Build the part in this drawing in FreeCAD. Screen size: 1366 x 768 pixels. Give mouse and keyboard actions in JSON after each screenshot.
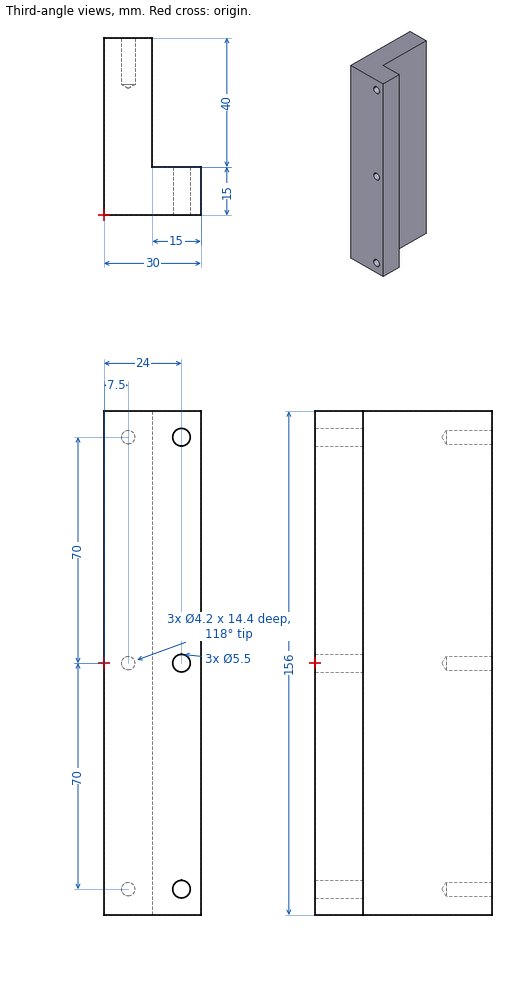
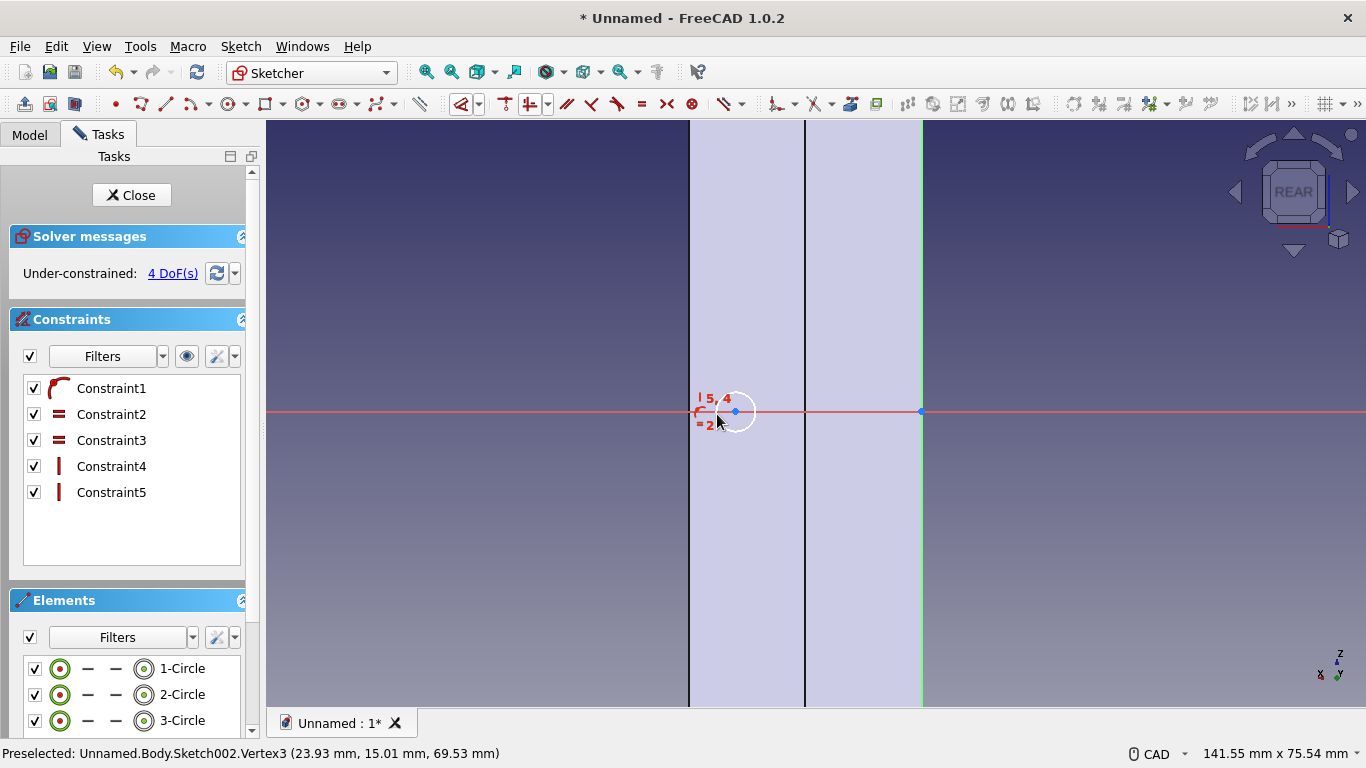
{"action": "left_click", "coordinate": [756, 413]}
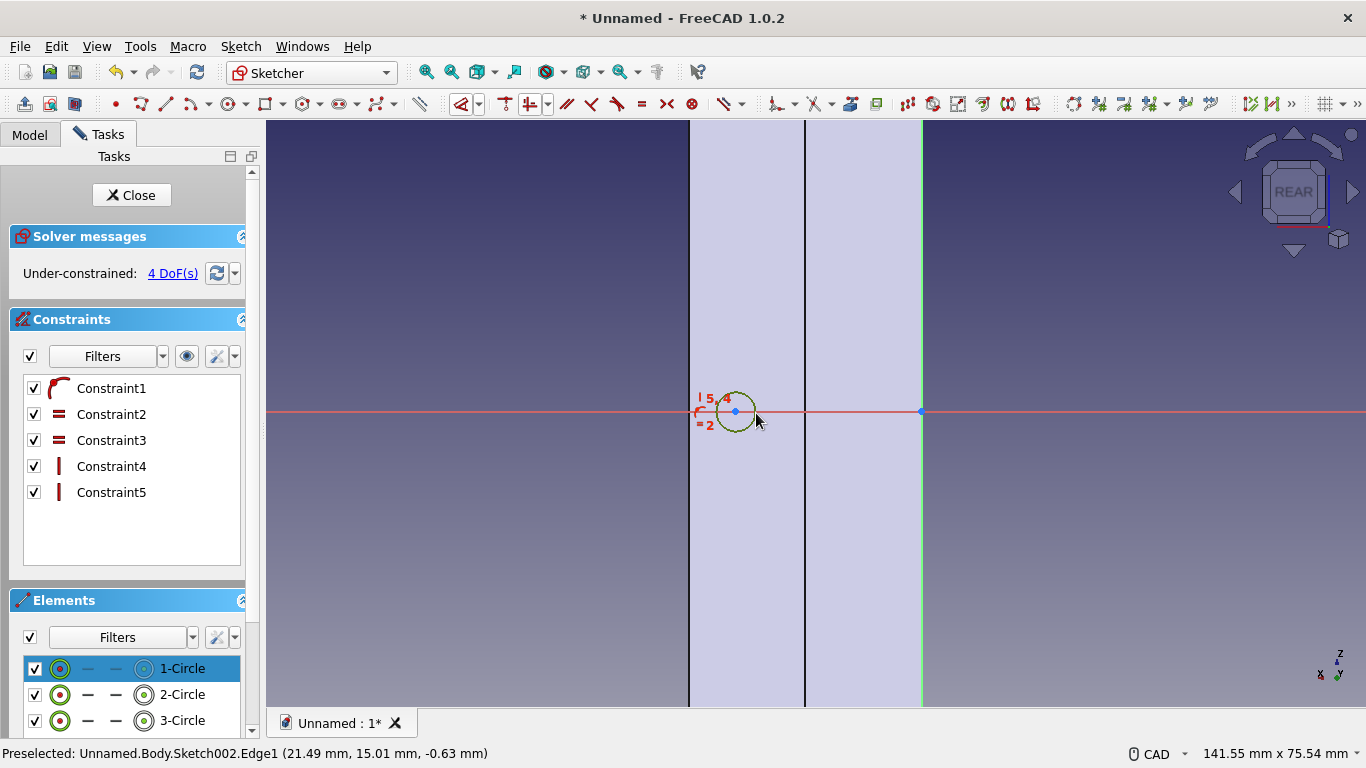
{"action": "key", "text": "k o"}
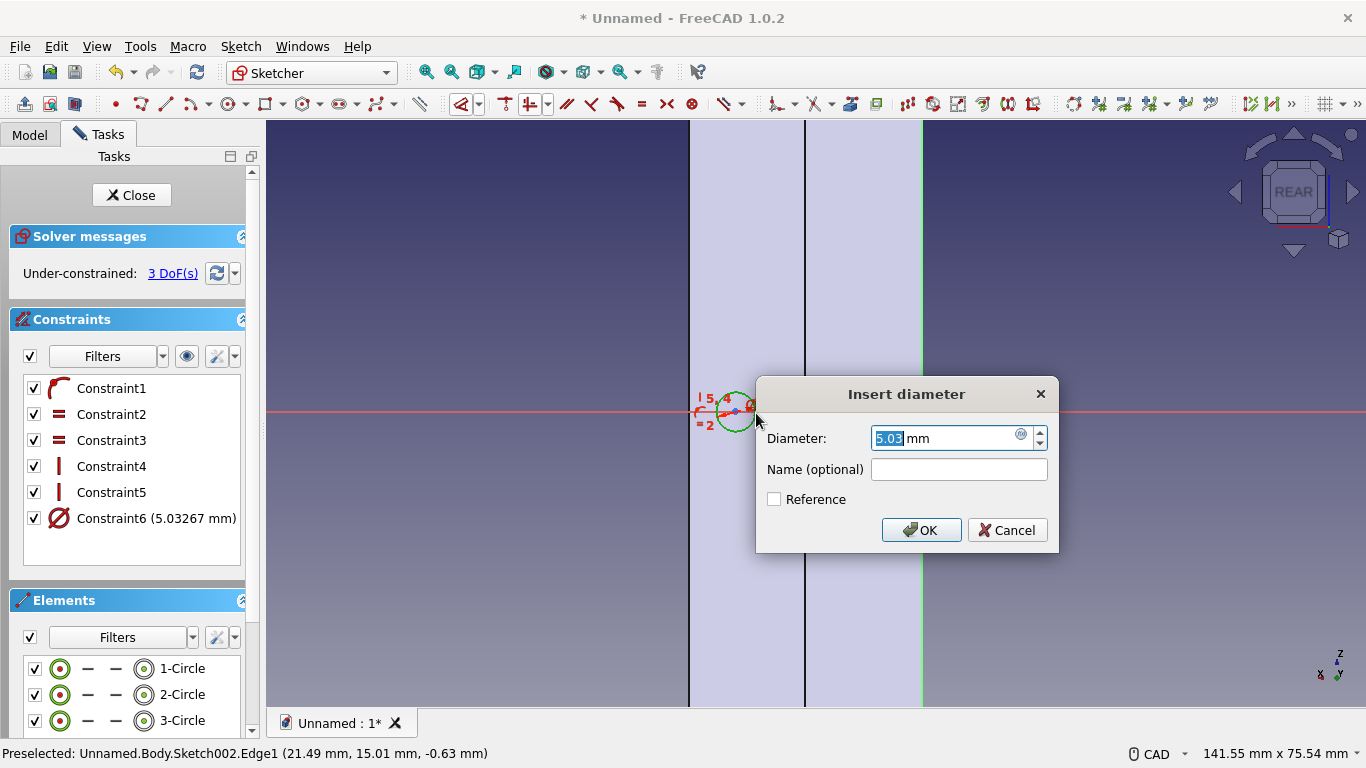
{"action": "type", "text": "5.5"}
{"action": "key", "text": "Return"}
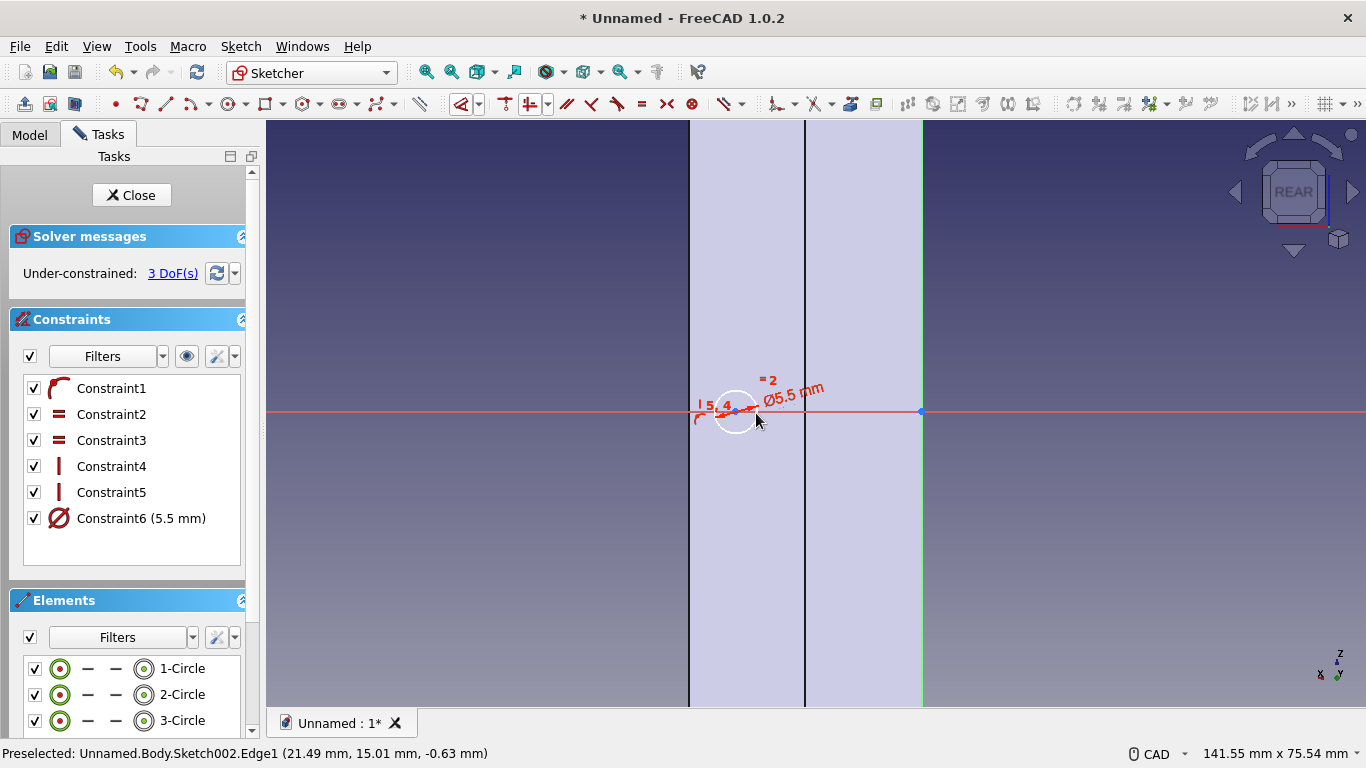
{"action": "left_click", "coordinate": [736, 412]}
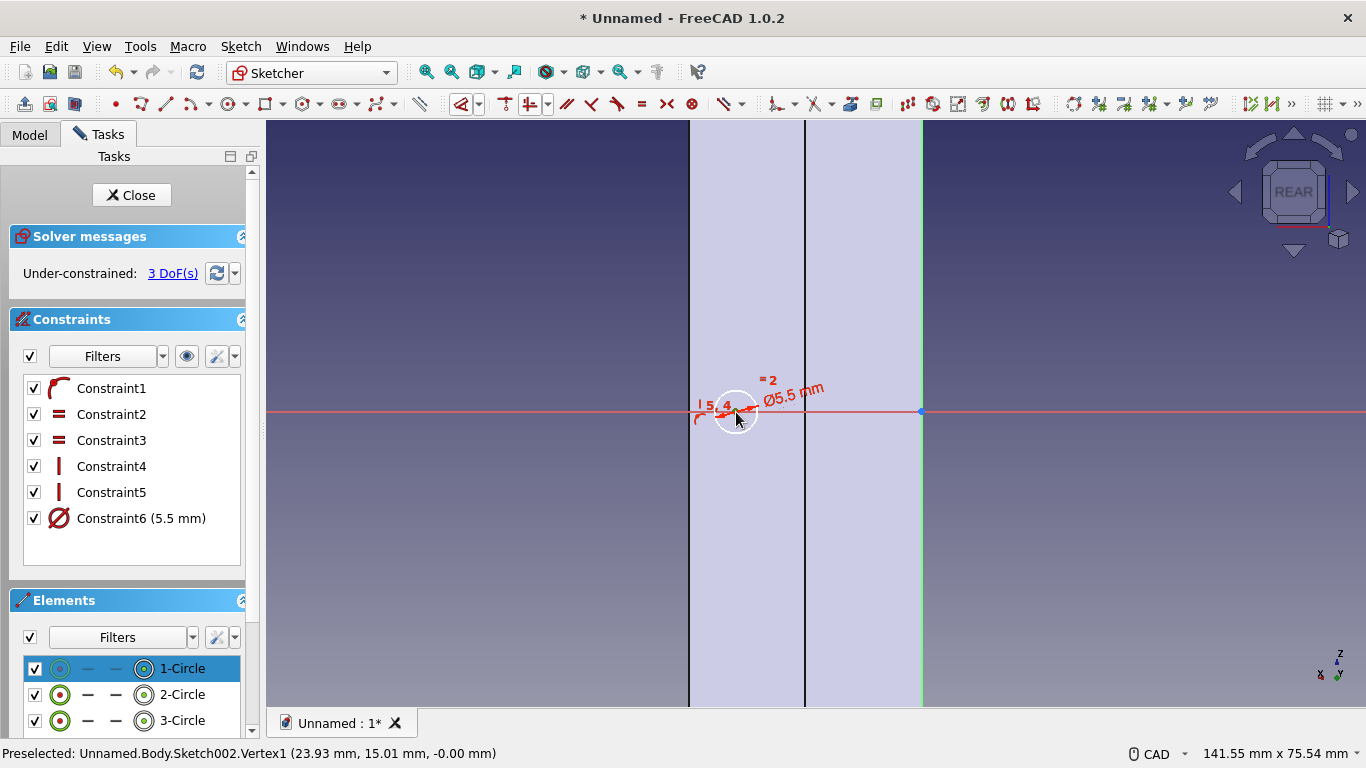
{"action": "key", "text": "l"}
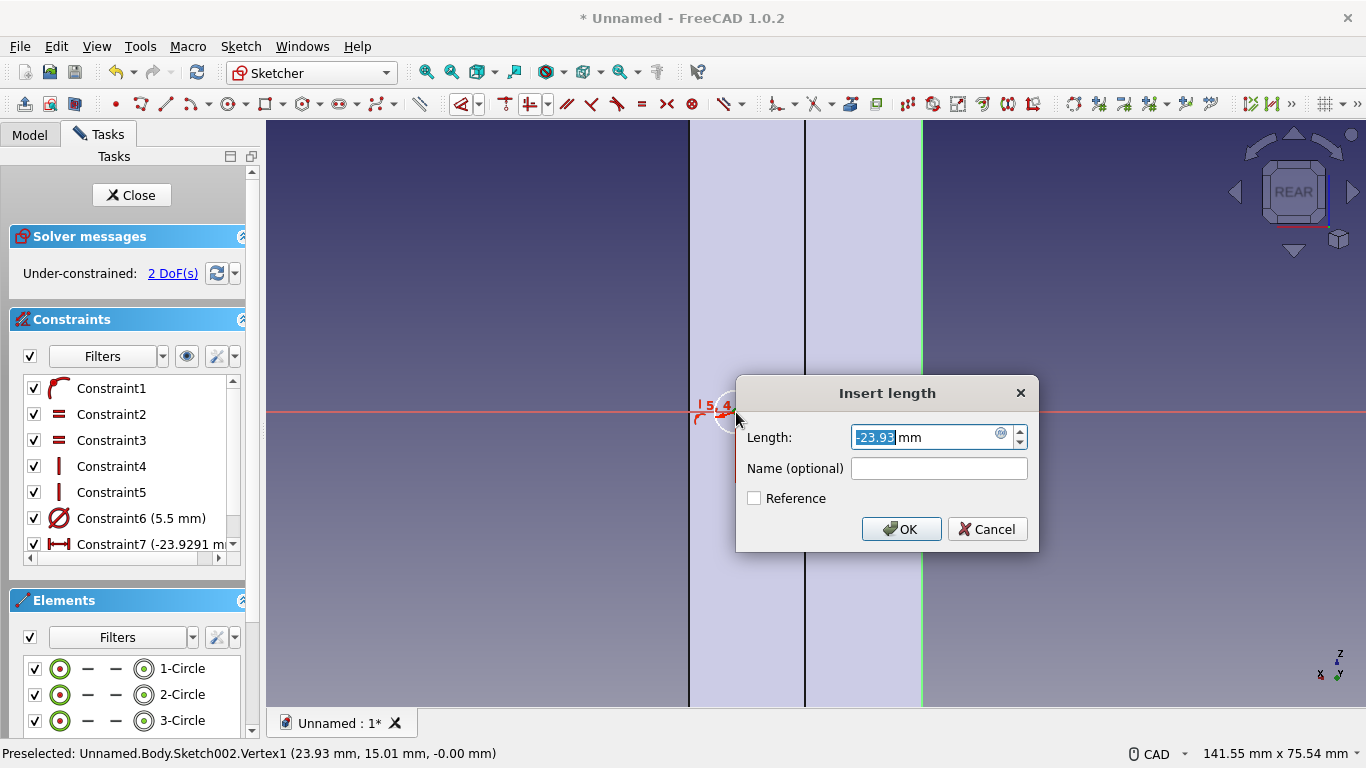
{"action": "type", "text": "-24"}
{"action": "key", "text": "Return"}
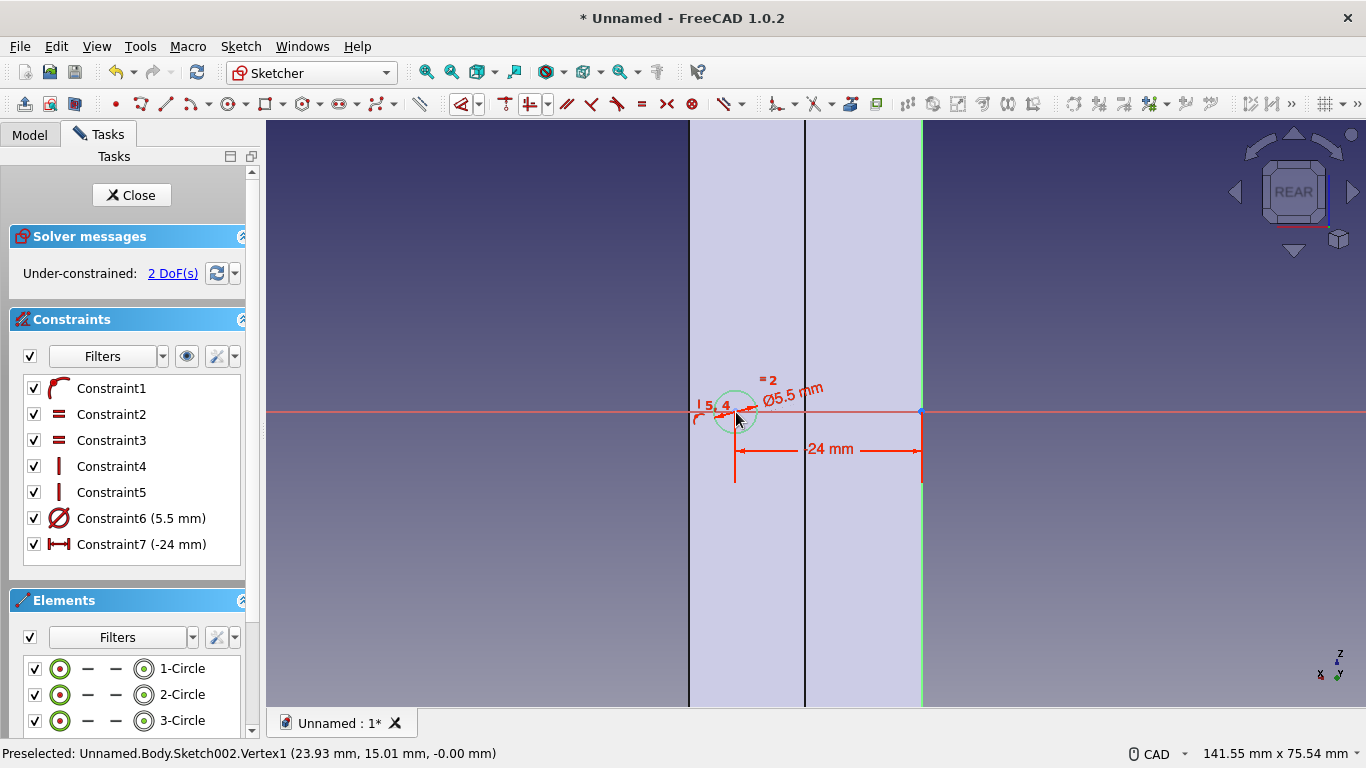
{"action": "scroll", "coordinate": [717, 414], "scroll_direction": "down", "scroll_amount": 6}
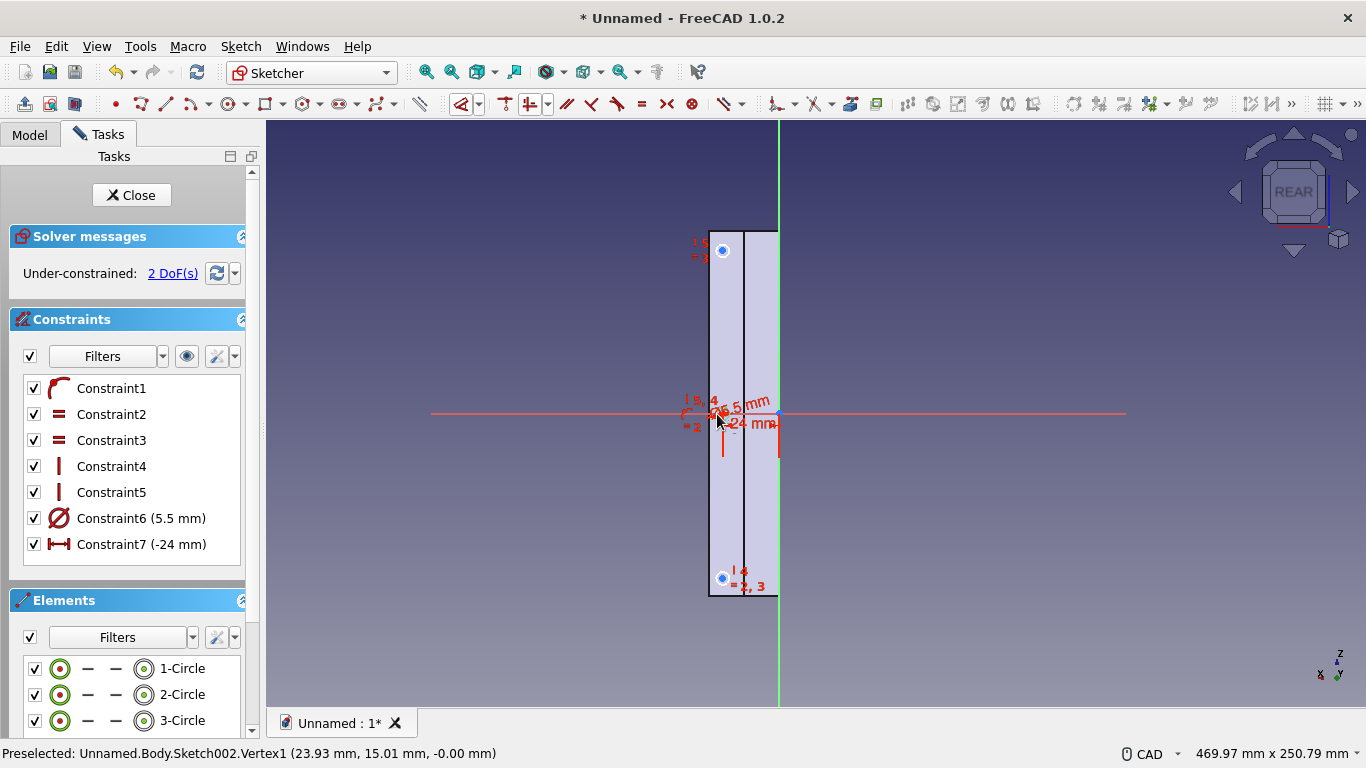
{"action": "left_click", "coordinate": [723, 578]}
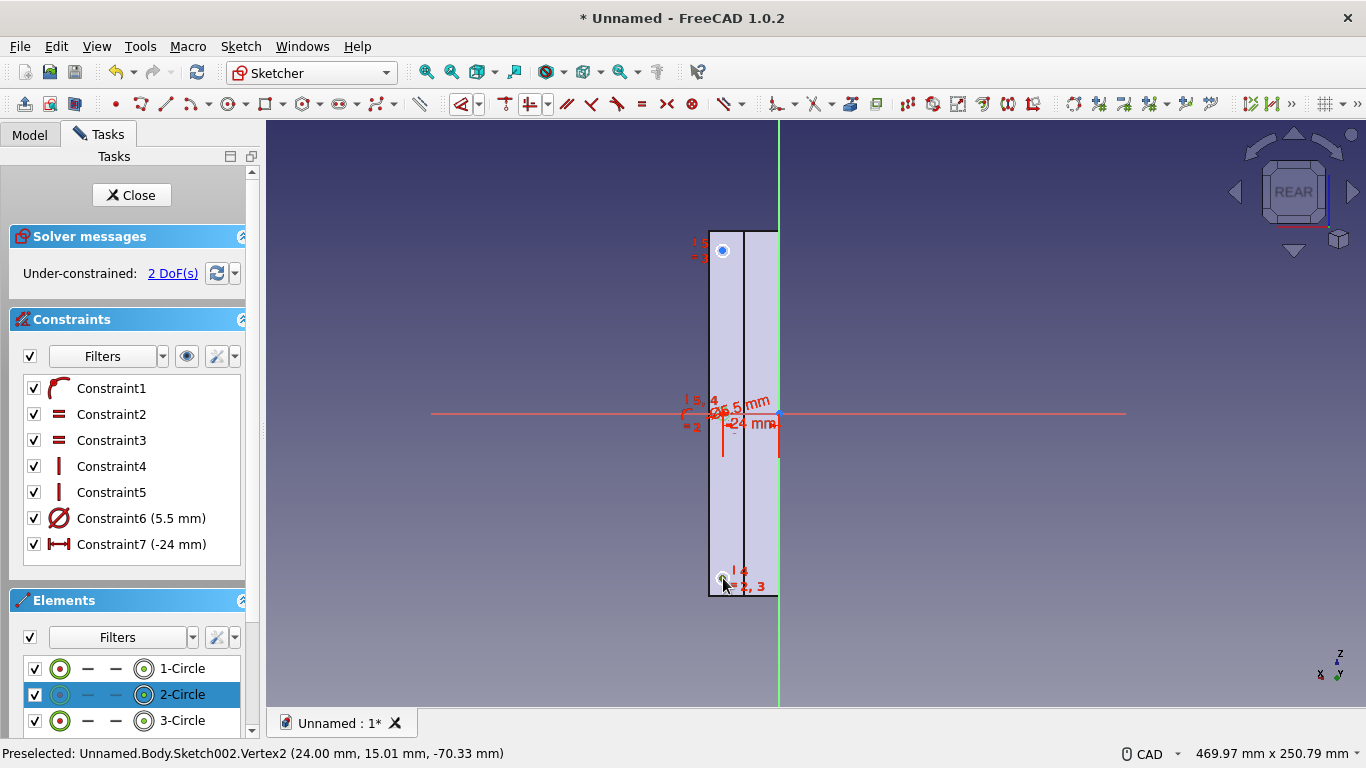
{"action": "key", "text": "i"}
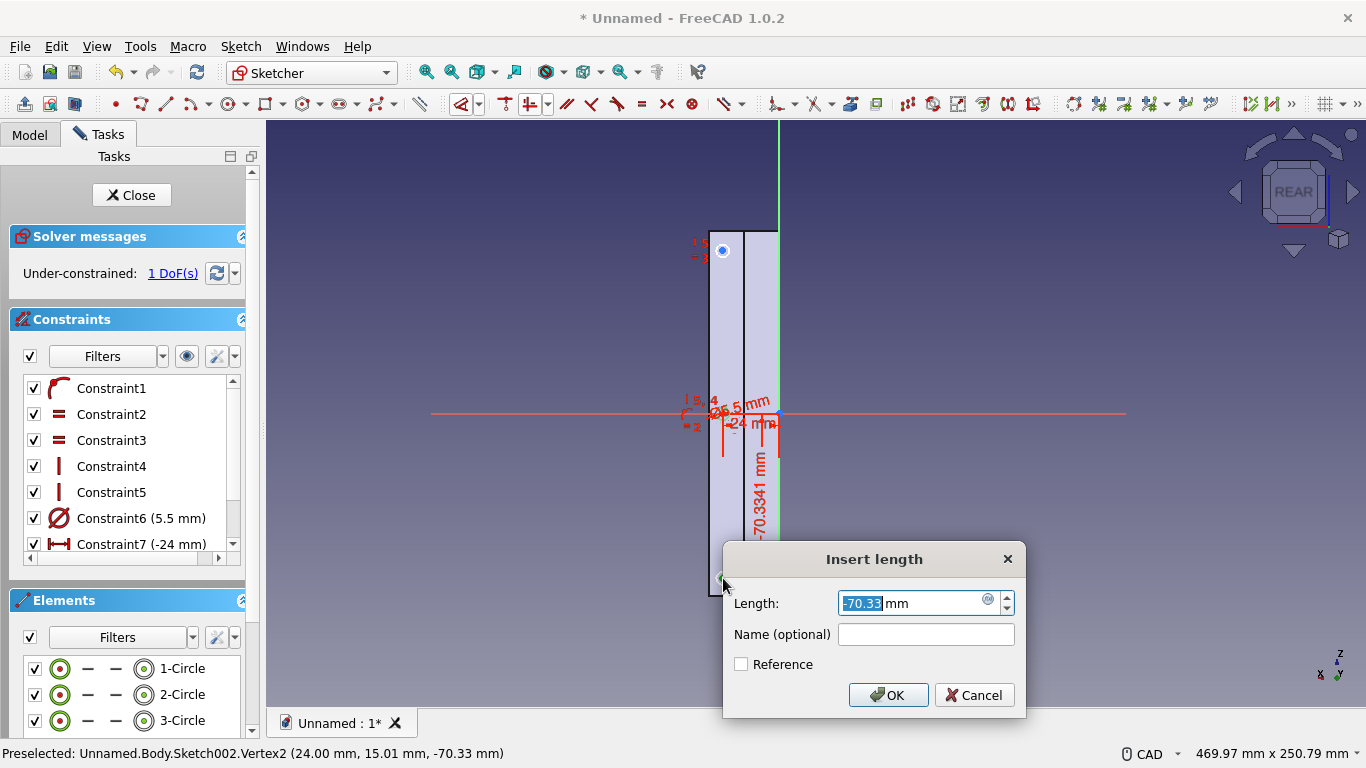
{"action": "type", "text": "-70"}
{"action": "key", "text": "Return"}